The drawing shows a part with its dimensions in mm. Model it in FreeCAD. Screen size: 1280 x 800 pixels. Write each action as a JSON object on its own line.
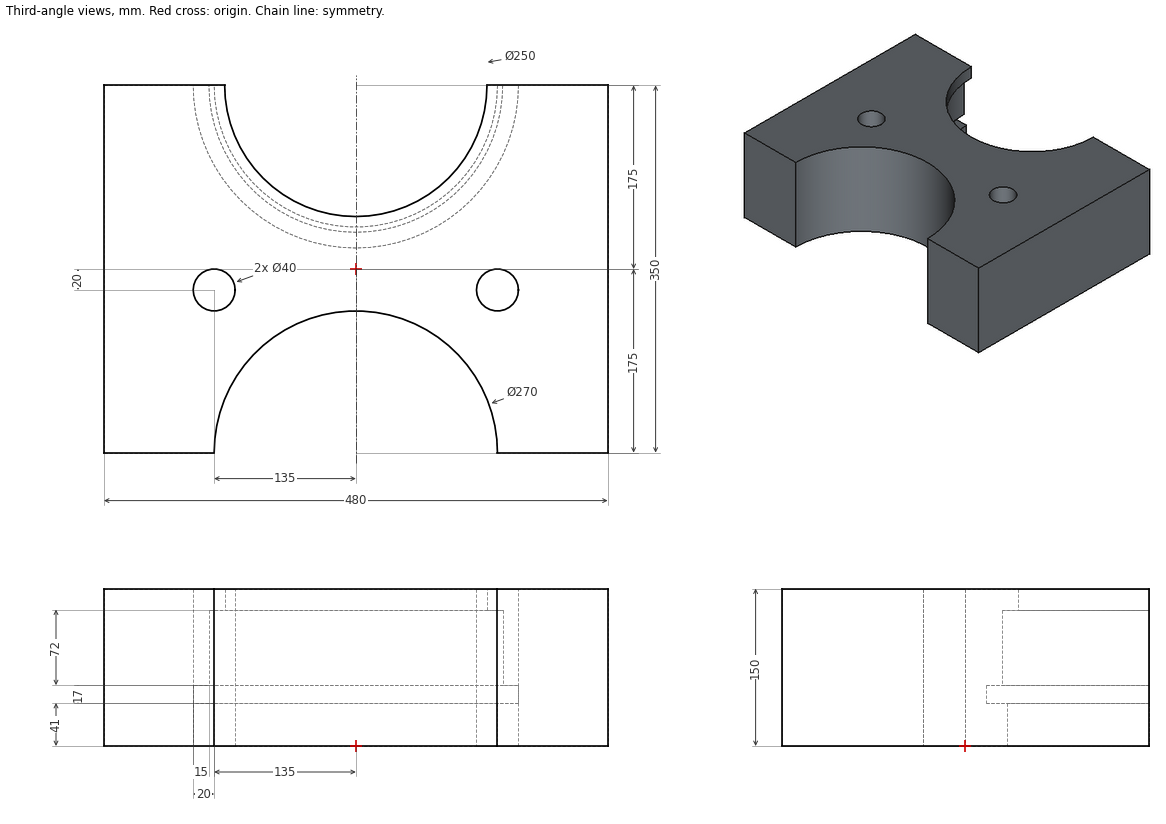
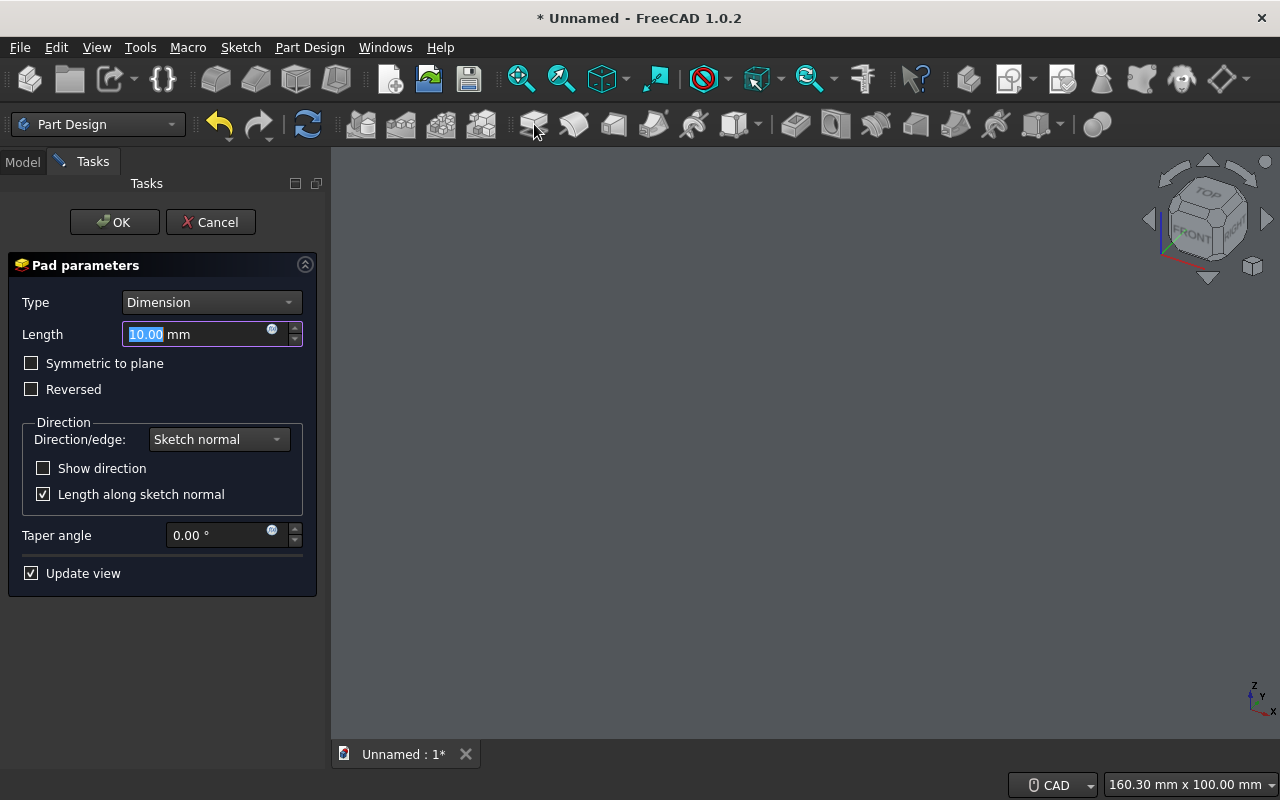
{"action": "type", "text": "150"}
{"action": "key", "text": "Tab"}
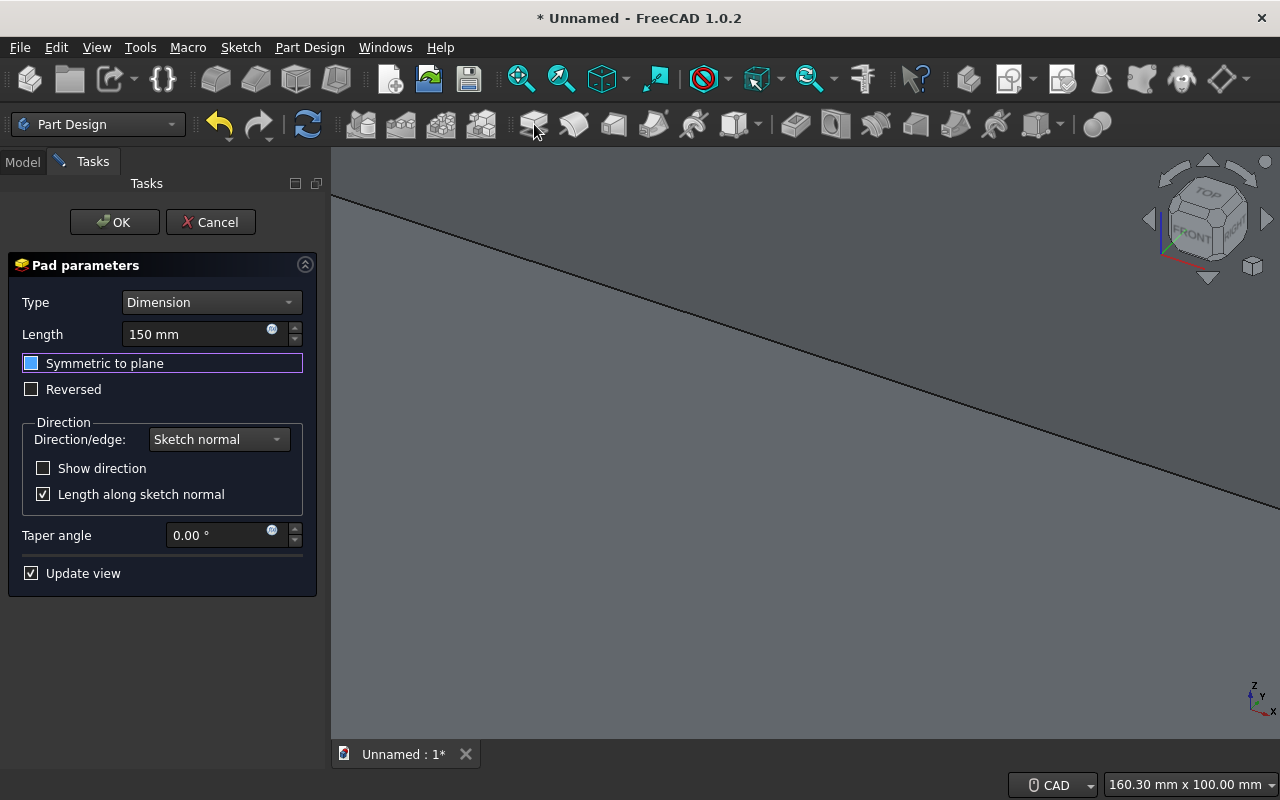
{"action": "left_click", "coordinate": [115, 222]}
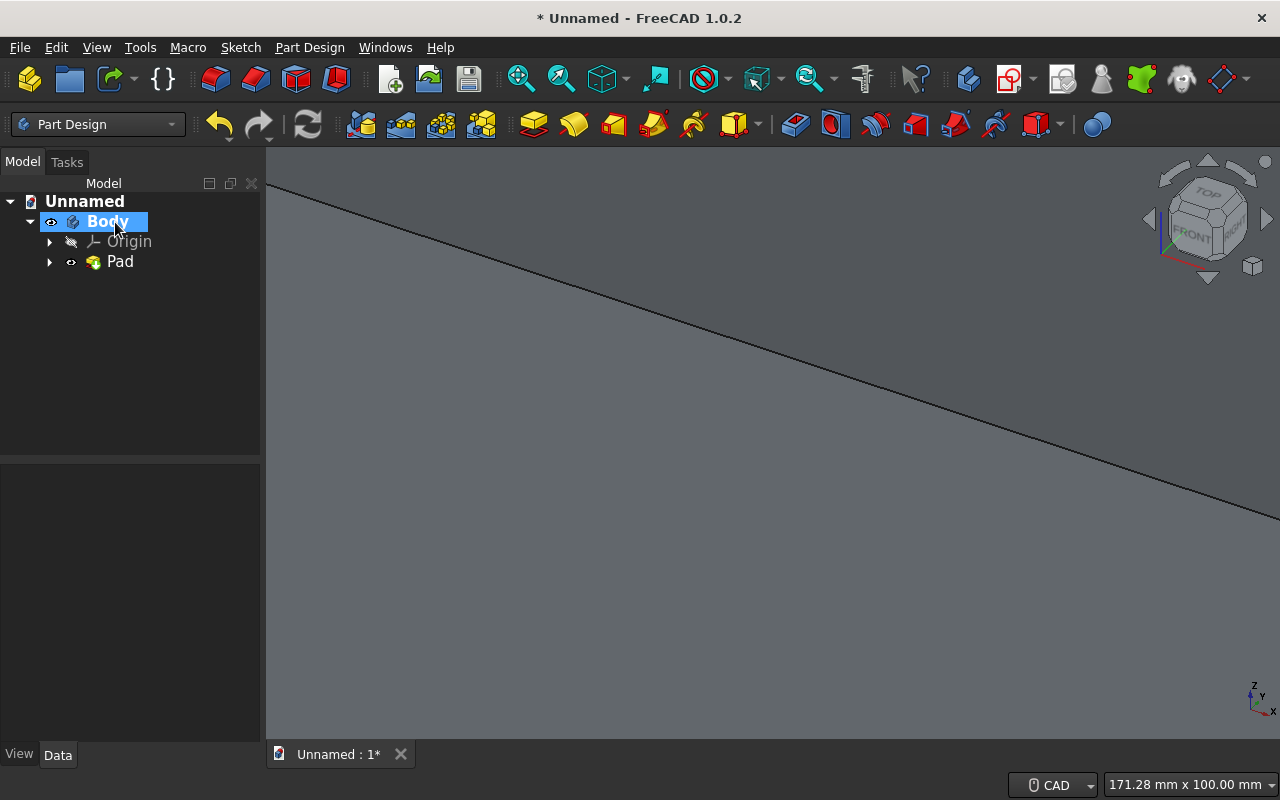
{"action": "left_click", "coordinate": [522, 80]}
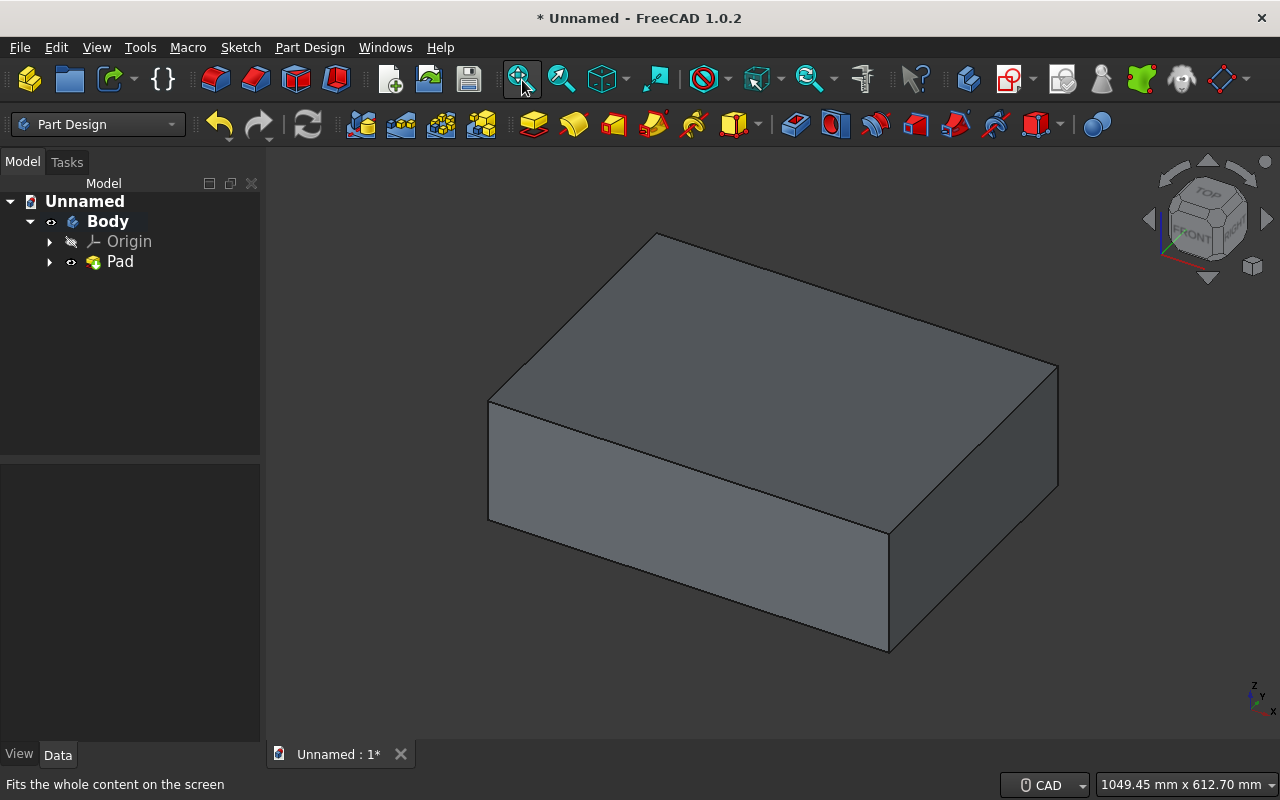
{"action": "left_click", "coordinate": [773, 383]}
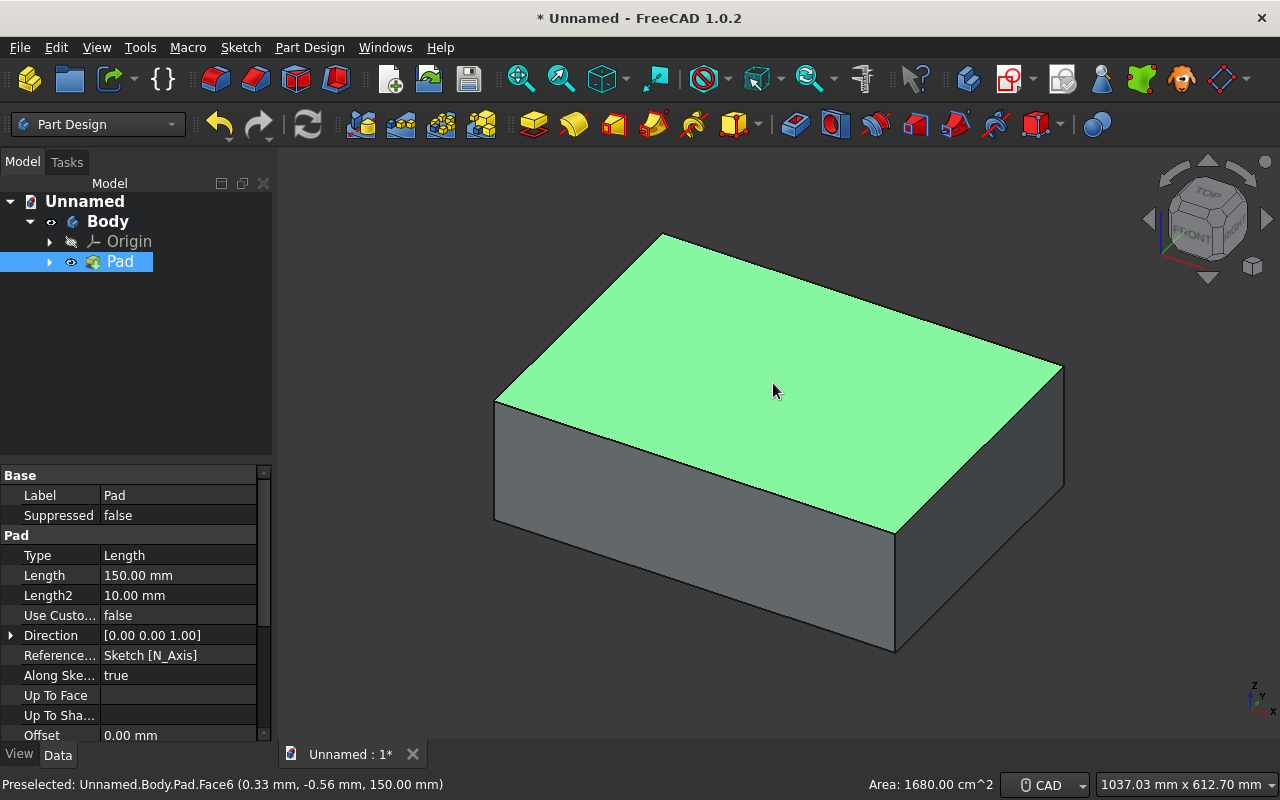
{"action": "left_click", "coordinate": [1010, 80]}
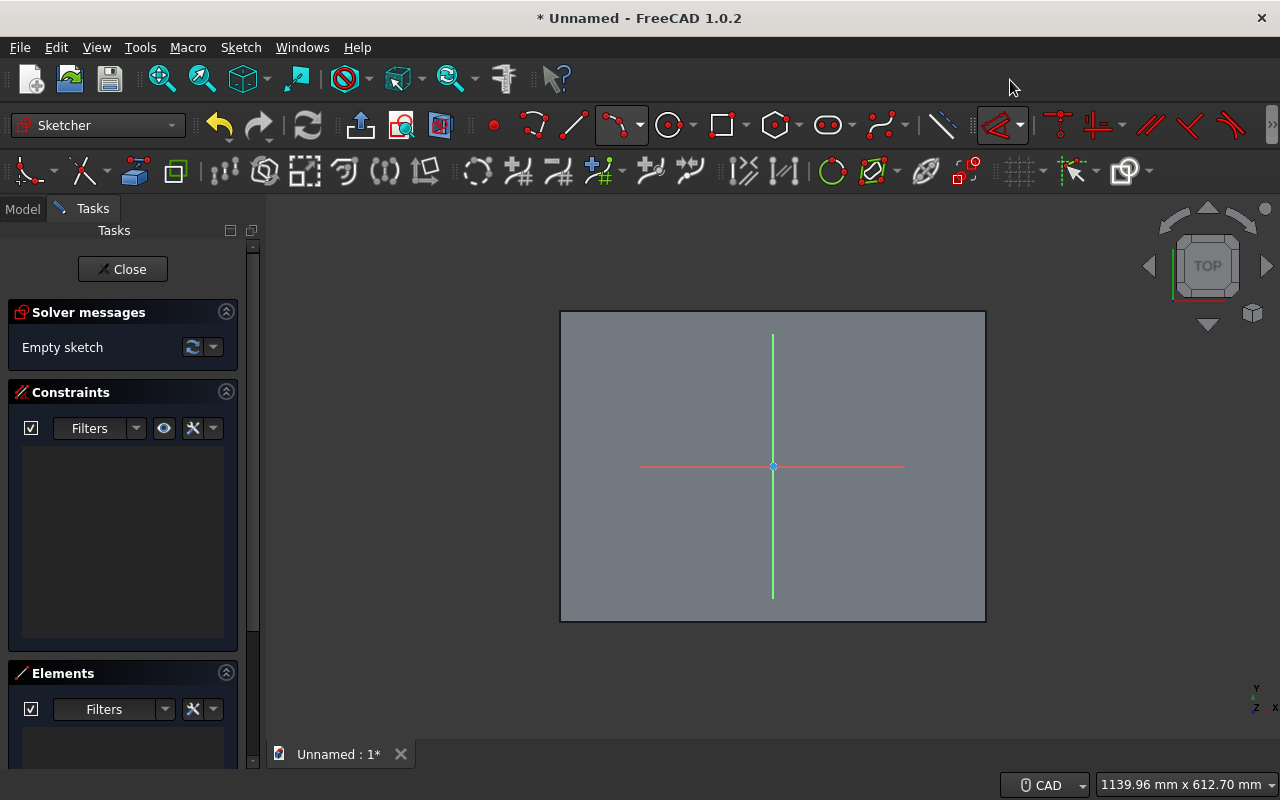
{"action": "scroll", "coordinate": [829, 499], "scroll_direction": "up", "scroll_amount": 4}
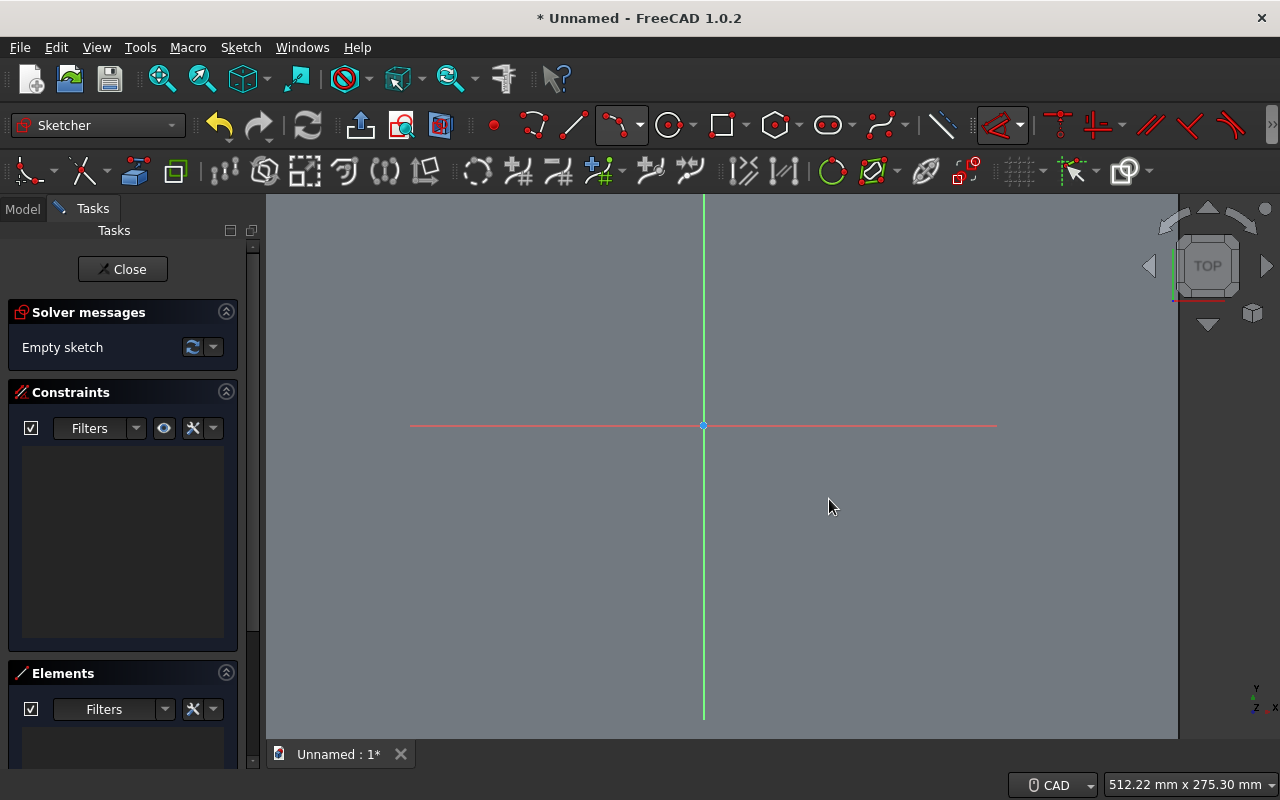
{"action": "key", "text": "g c"}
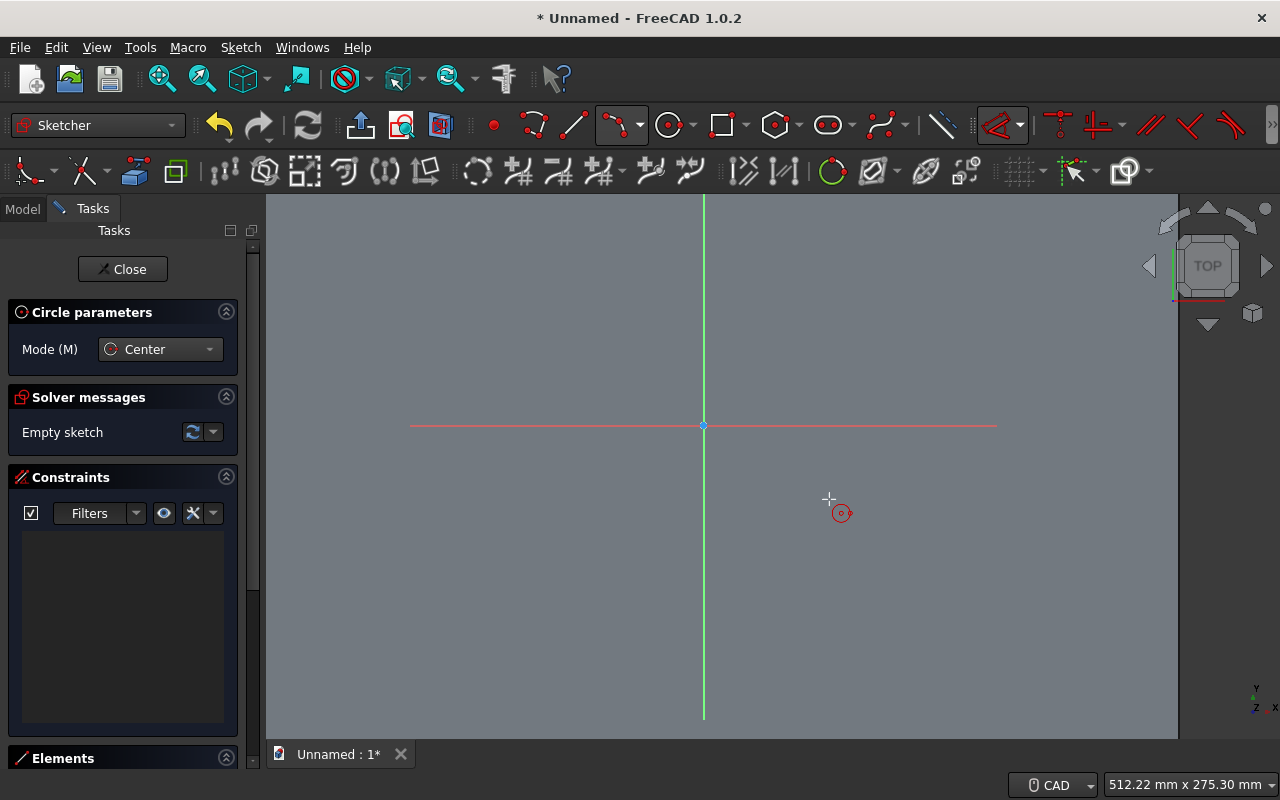
{"action": "left_click", "coordinate": [436, 466]}
{"action": "mouse_move", "coordinate": [464, 494]}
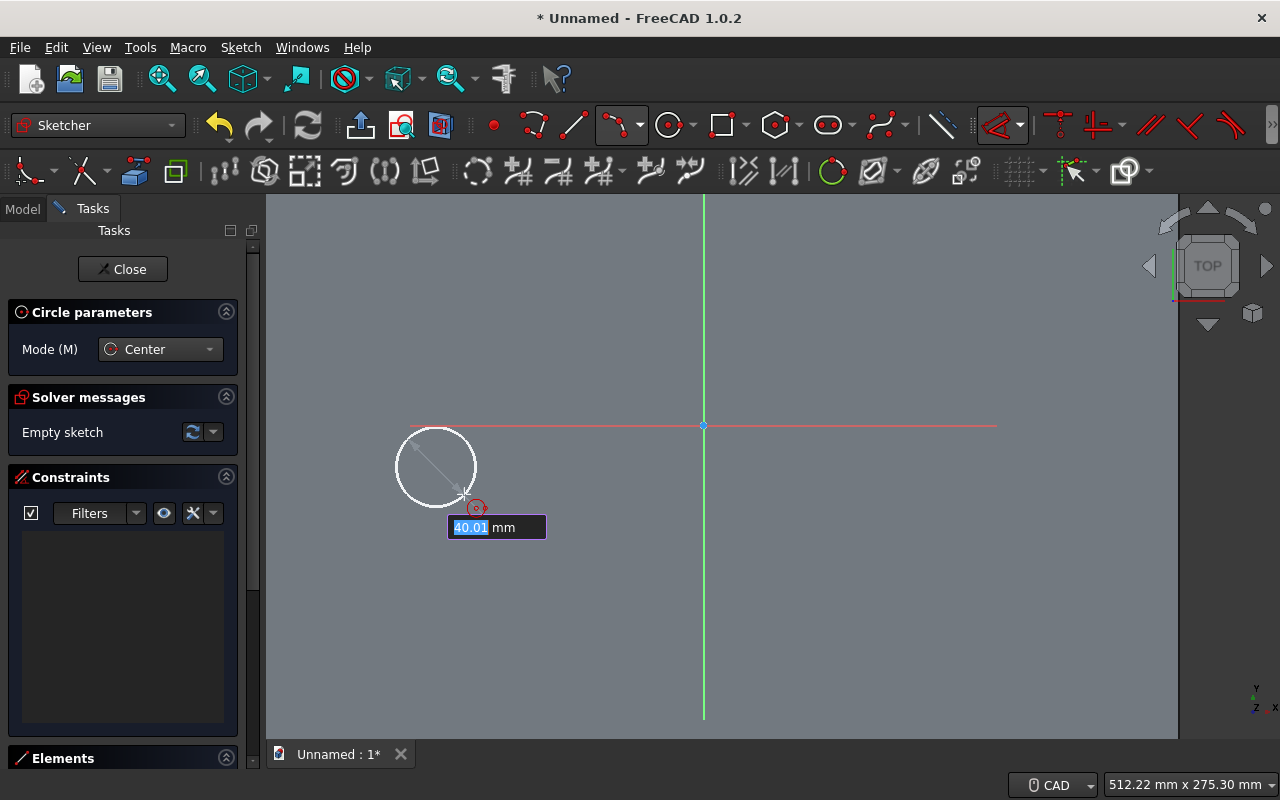
{"action": "type", "text": "40"}
{"action": "key", "text": "Return"}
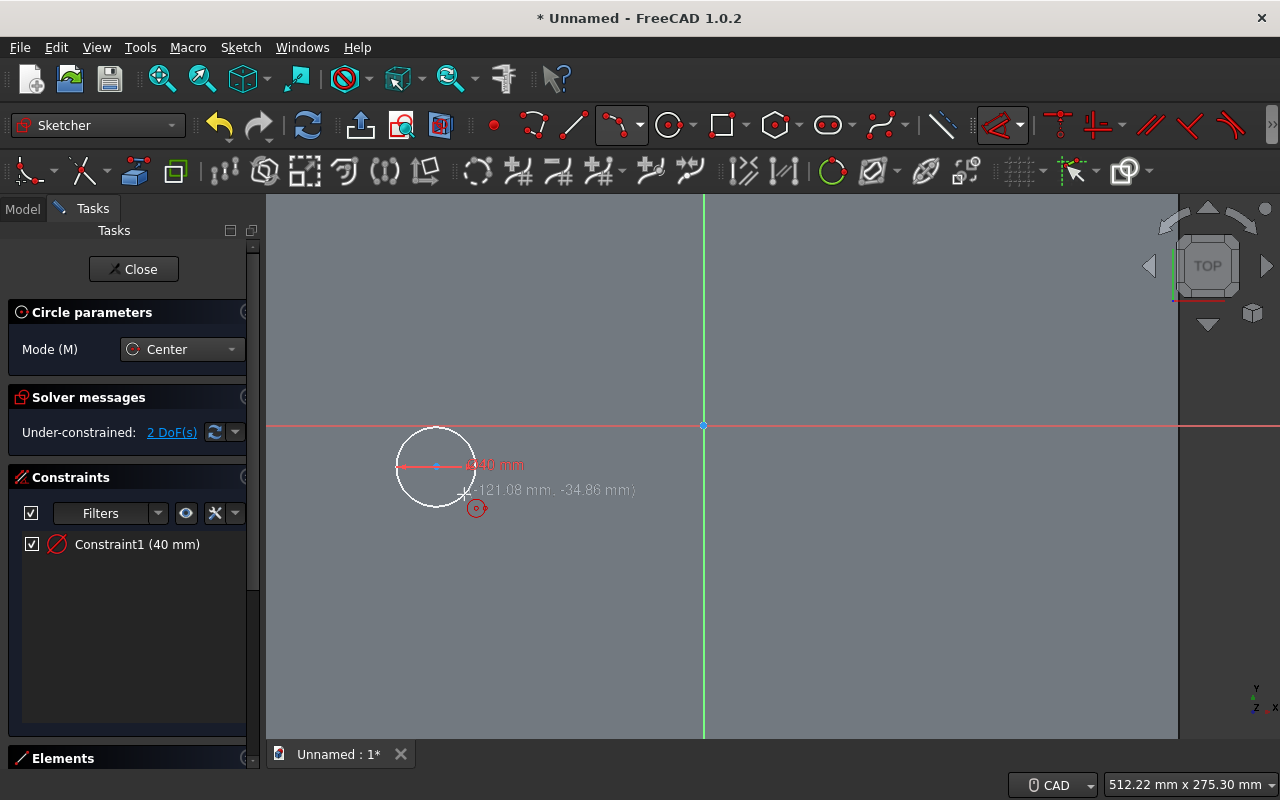
{"action": "left_click", "coordinate": [971, 466]}
{"action": "mouse_move", "coordinate": [999, 494]}